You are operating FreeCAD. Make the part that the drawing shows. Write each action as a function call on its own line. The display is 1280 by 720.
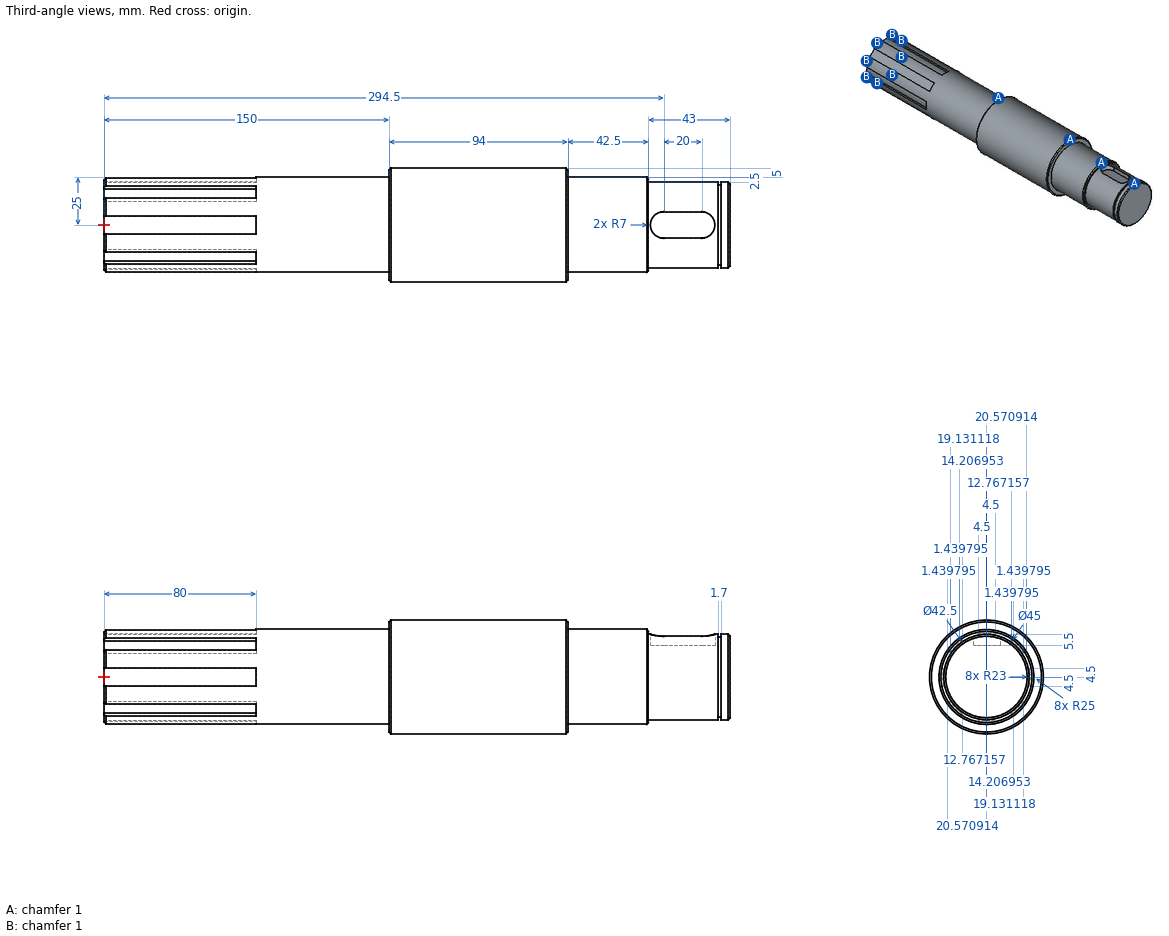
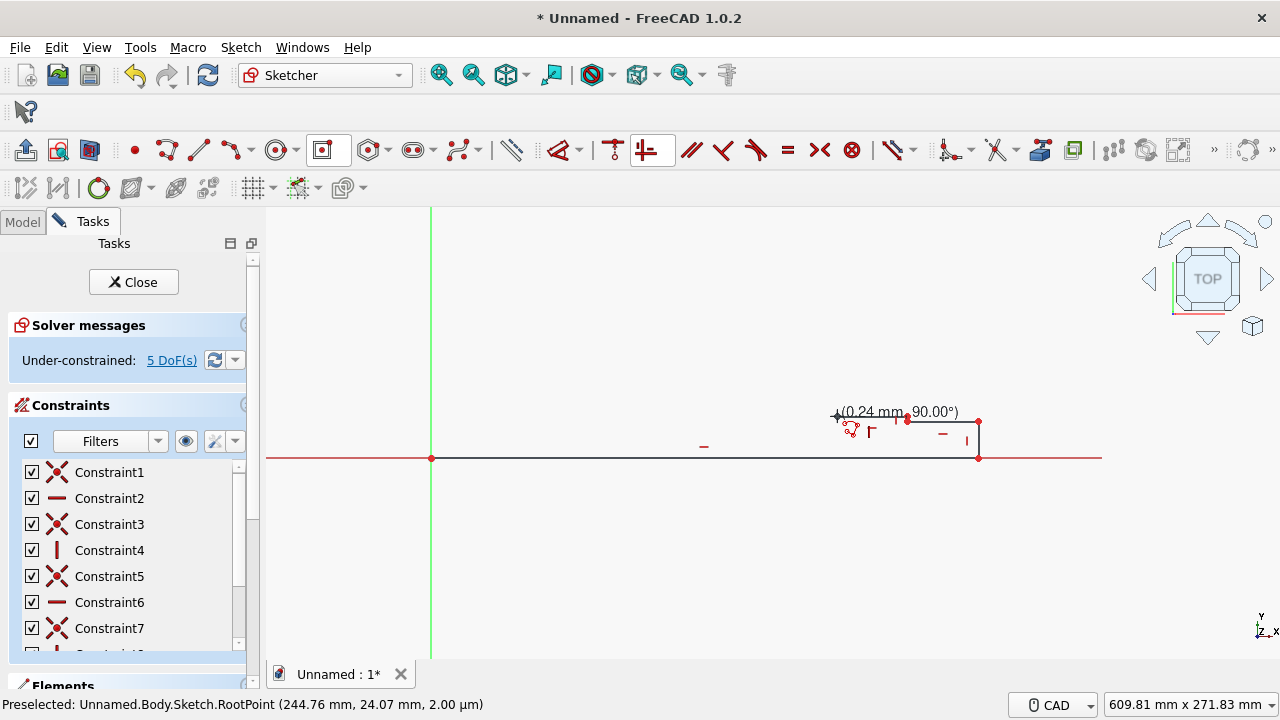
scroll(837, 408, up, 4)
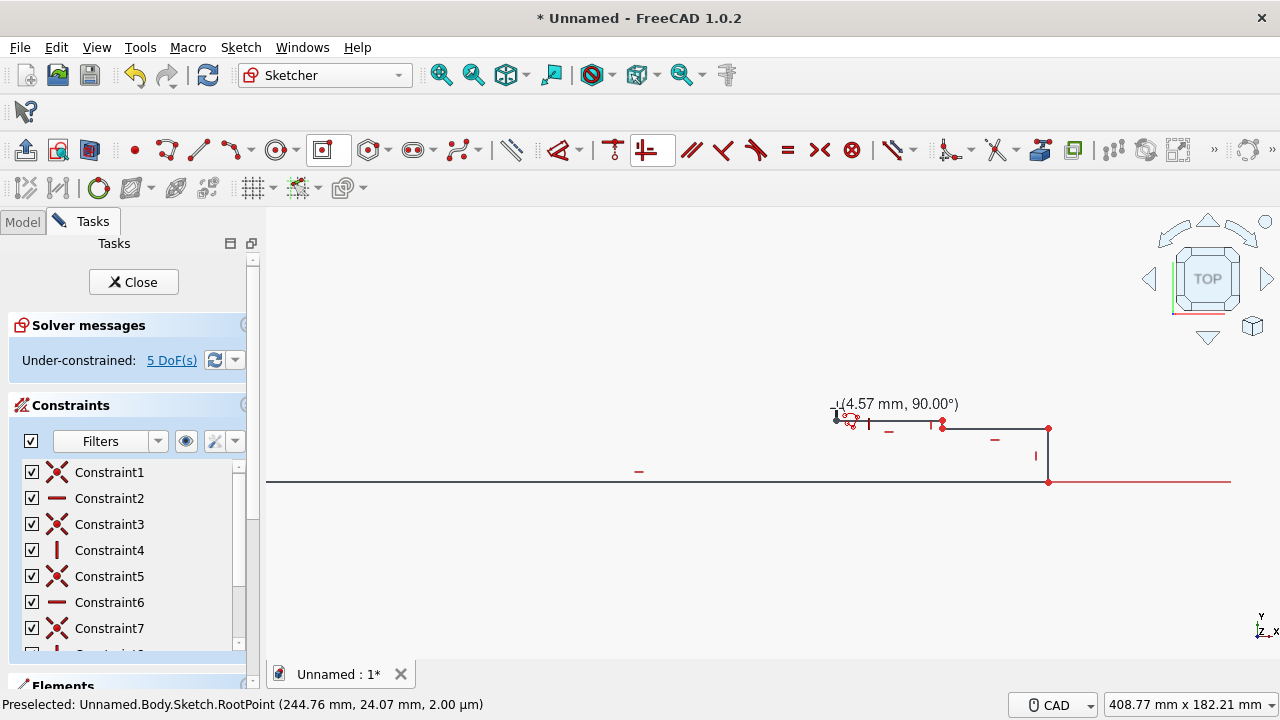
click(836, 408)
click(488, 408)
click(488, 426)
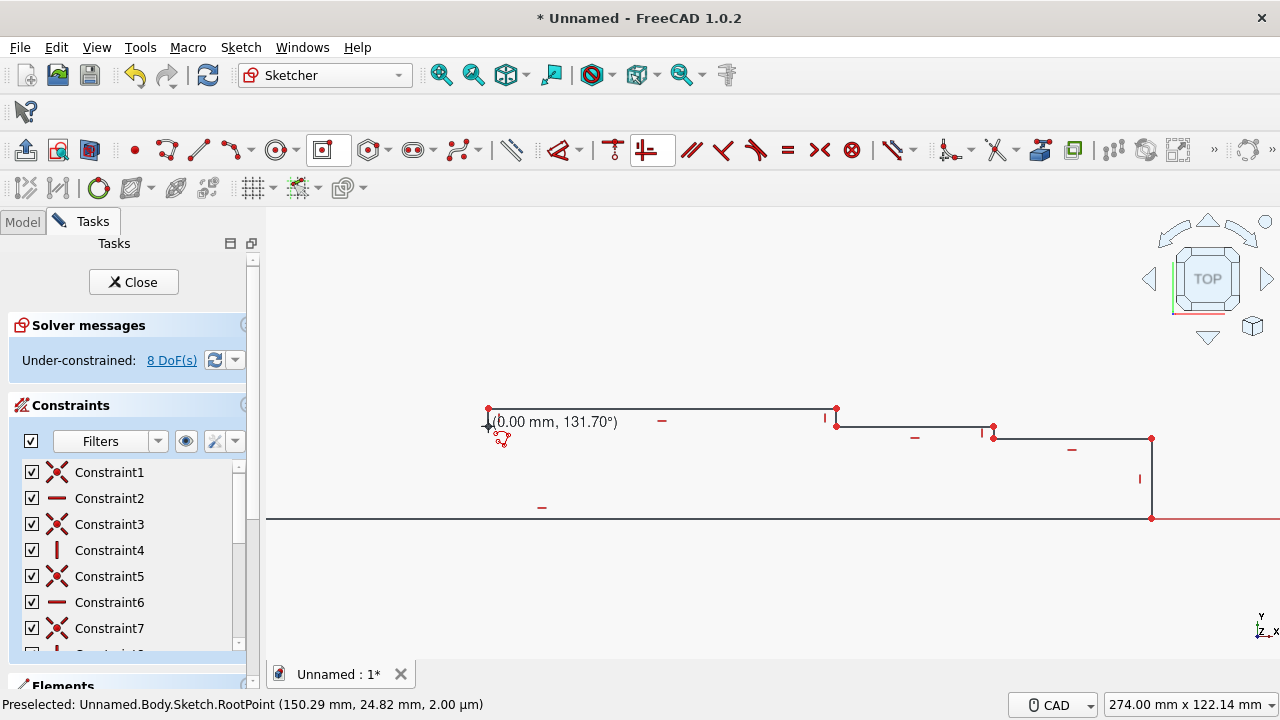
scroll(837, 408, down, 4)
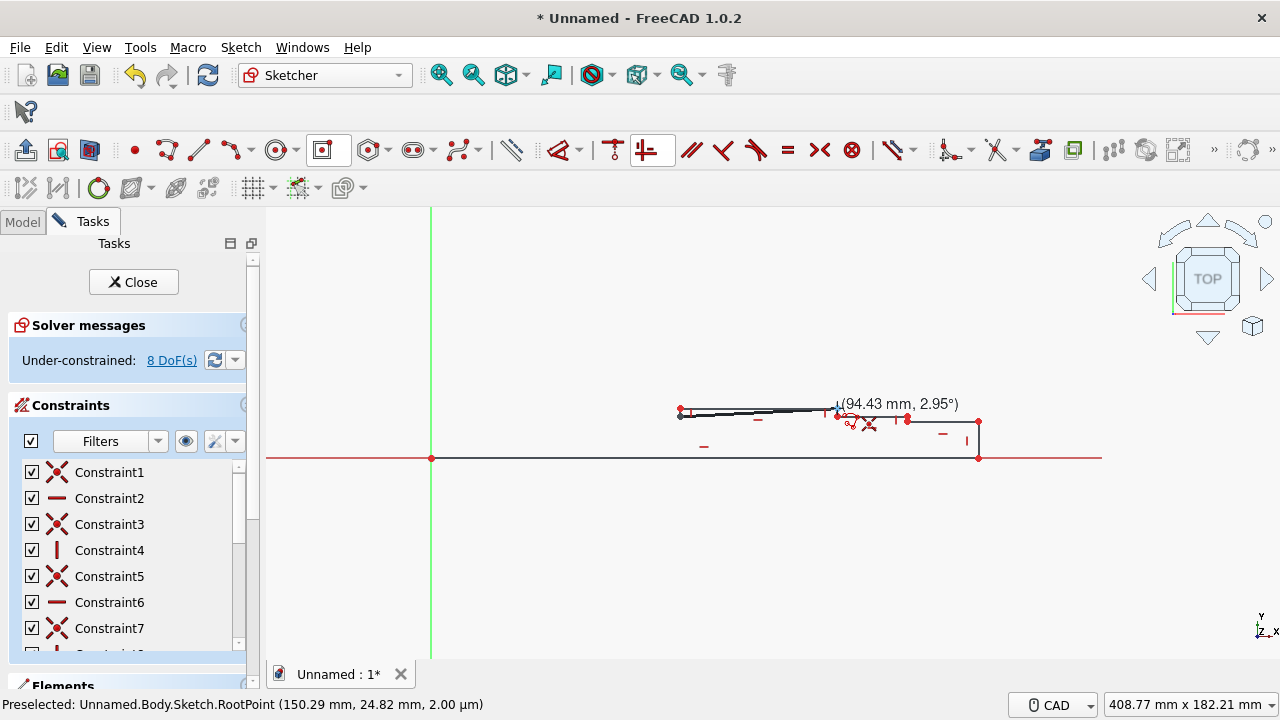
click(440, 416)
click(431, 458)
key(Escape)
key(Escape)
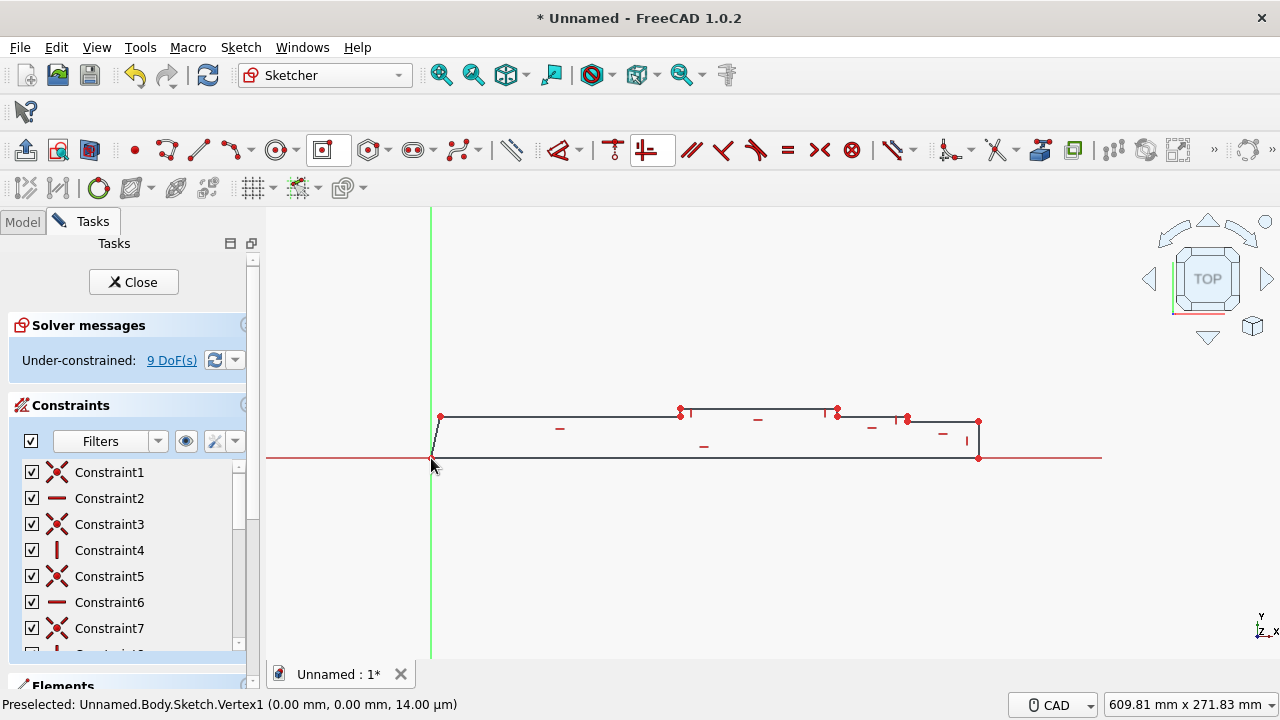
click(434, 446)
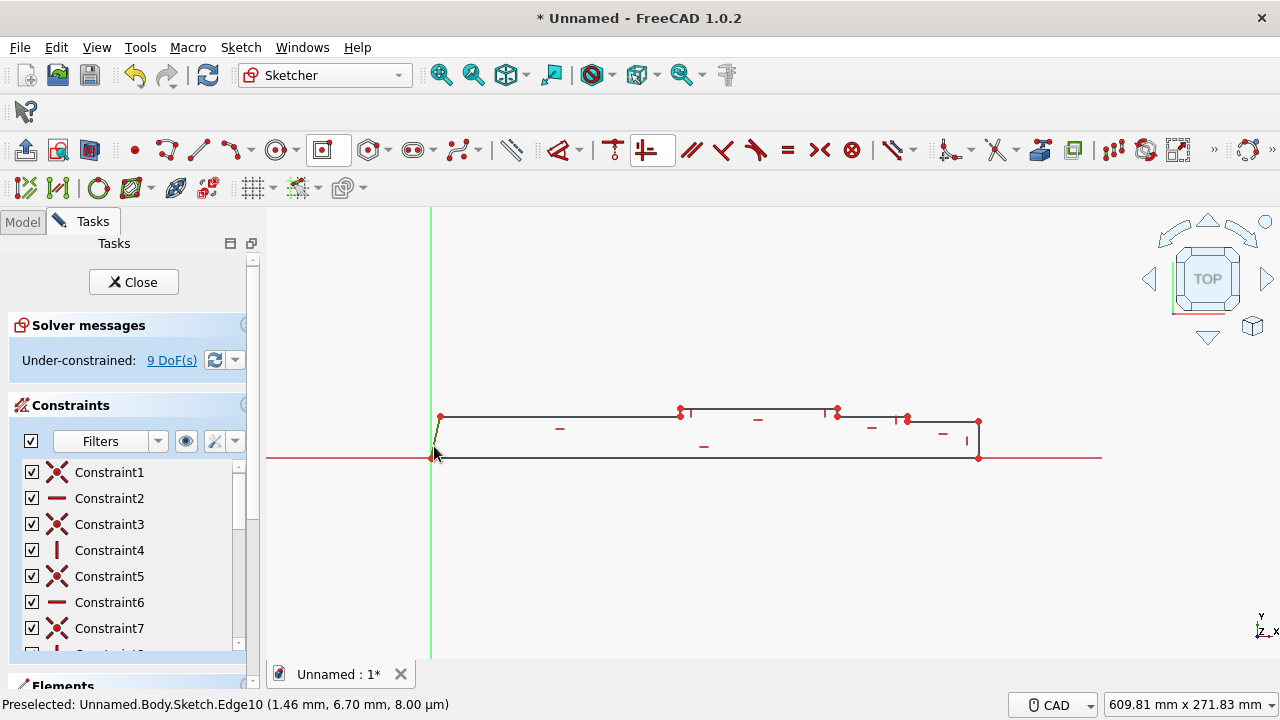
key(v)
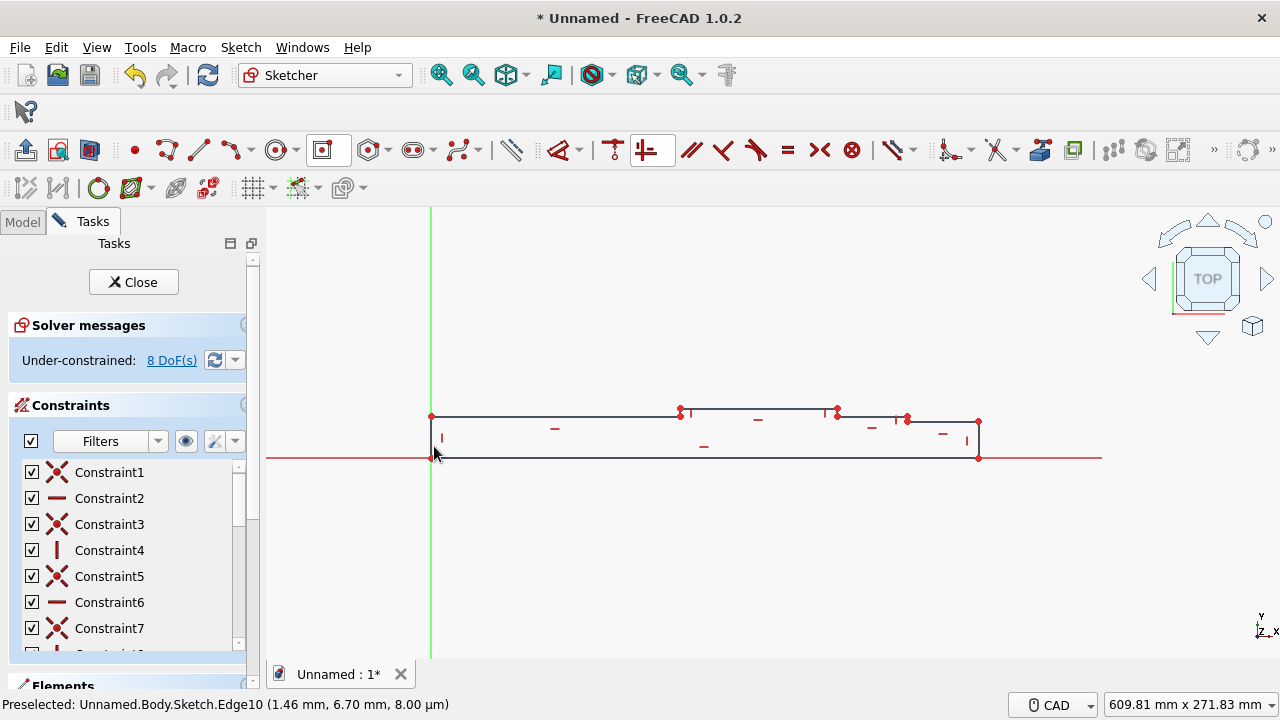
click(558, 150)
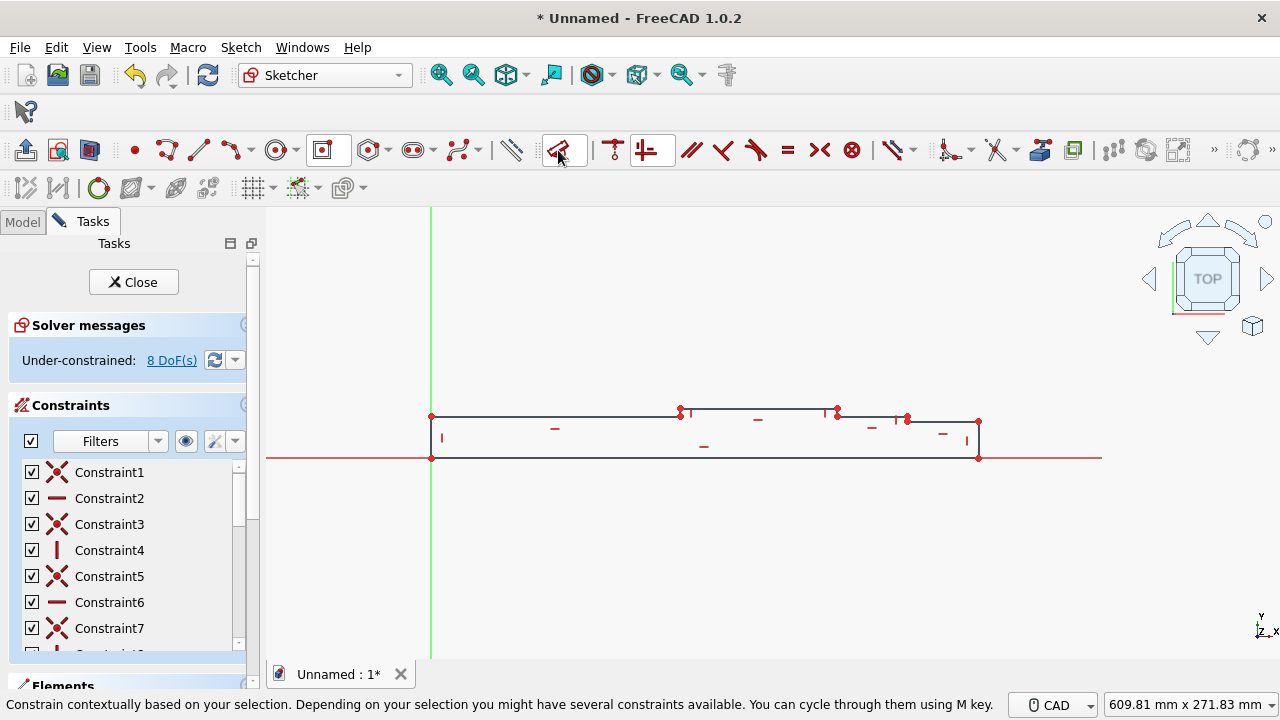
scroll(837, 413, up, 8)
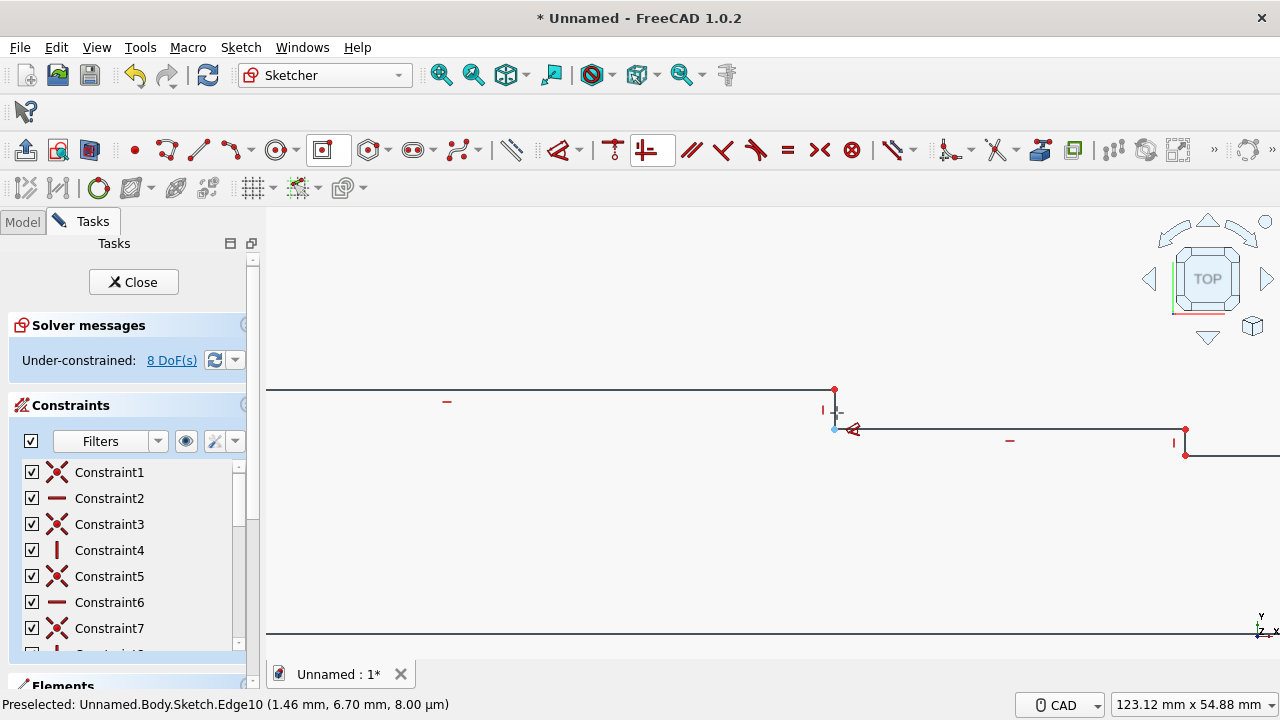
click(835, 409)
click(869, 409)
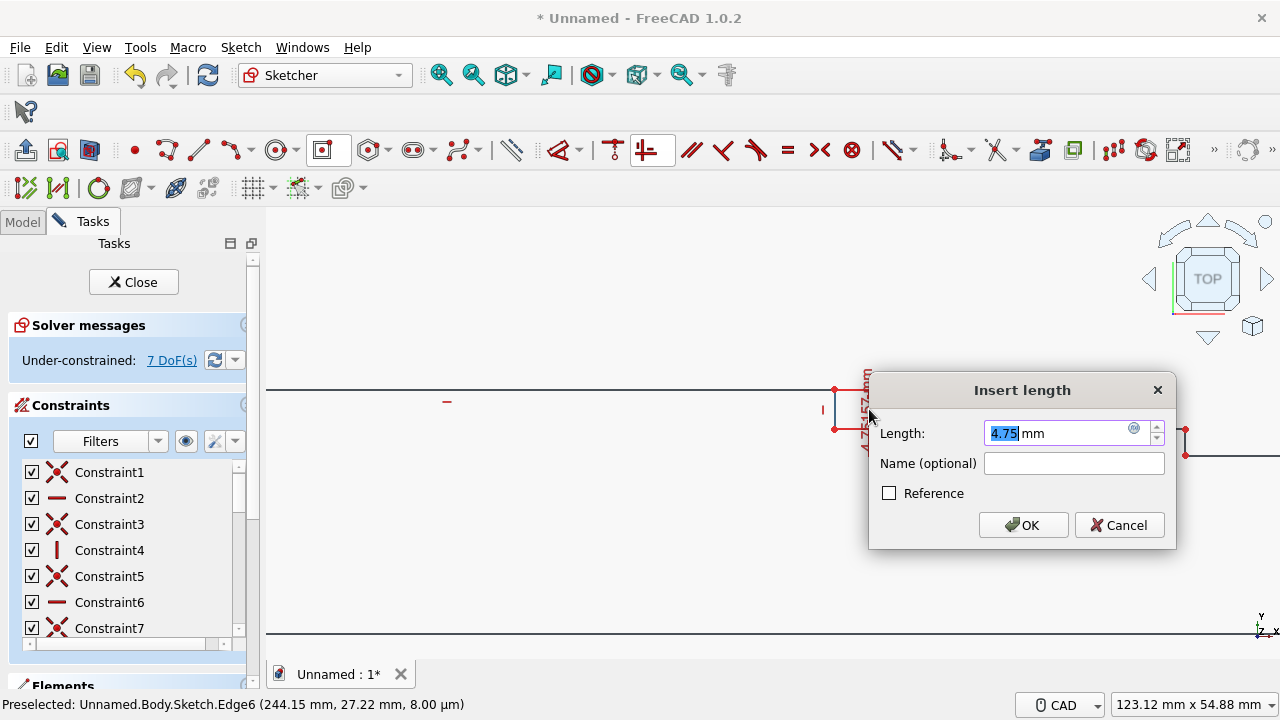
text(5)
key(Return)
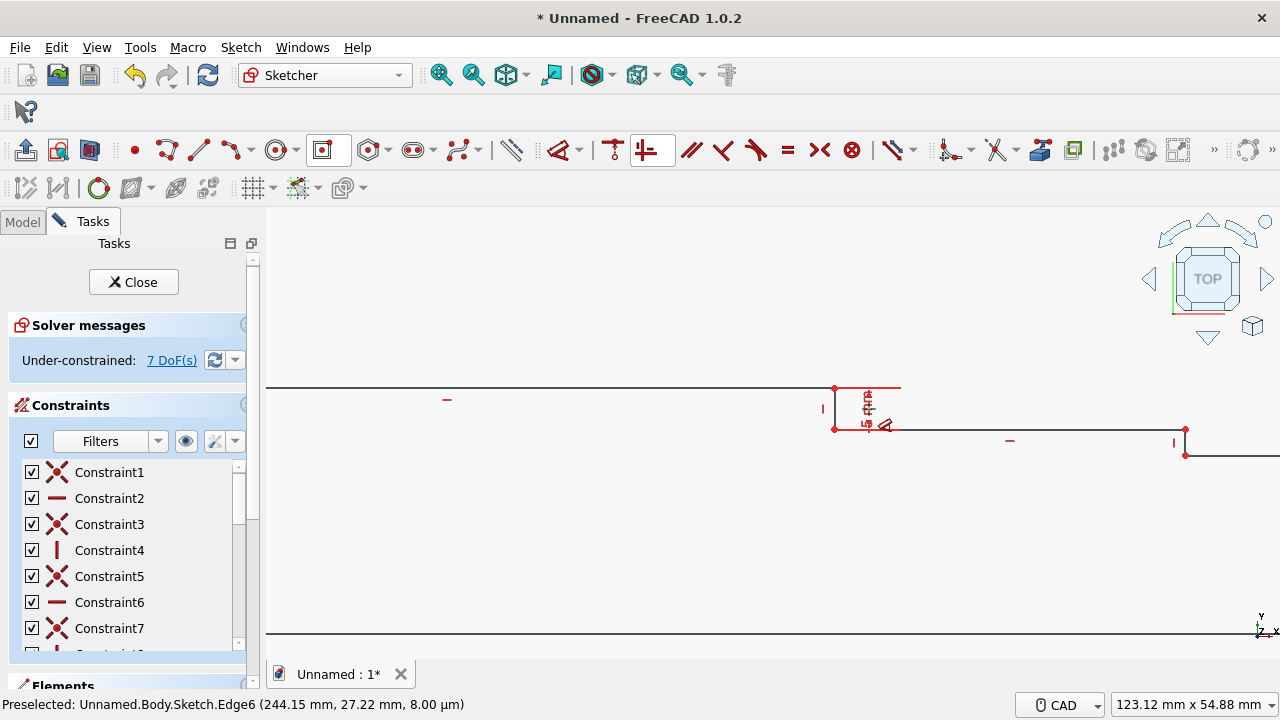
scroll(837, 413, down, 8)